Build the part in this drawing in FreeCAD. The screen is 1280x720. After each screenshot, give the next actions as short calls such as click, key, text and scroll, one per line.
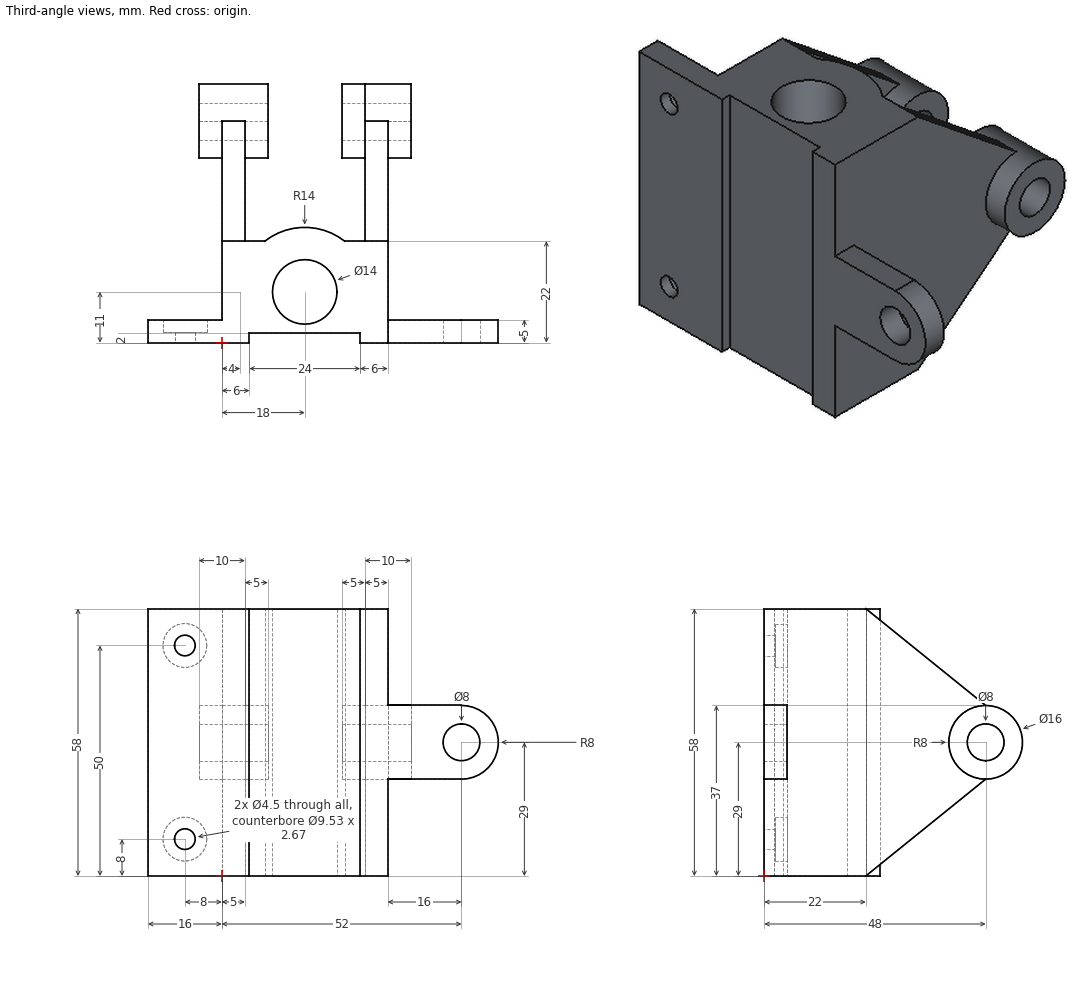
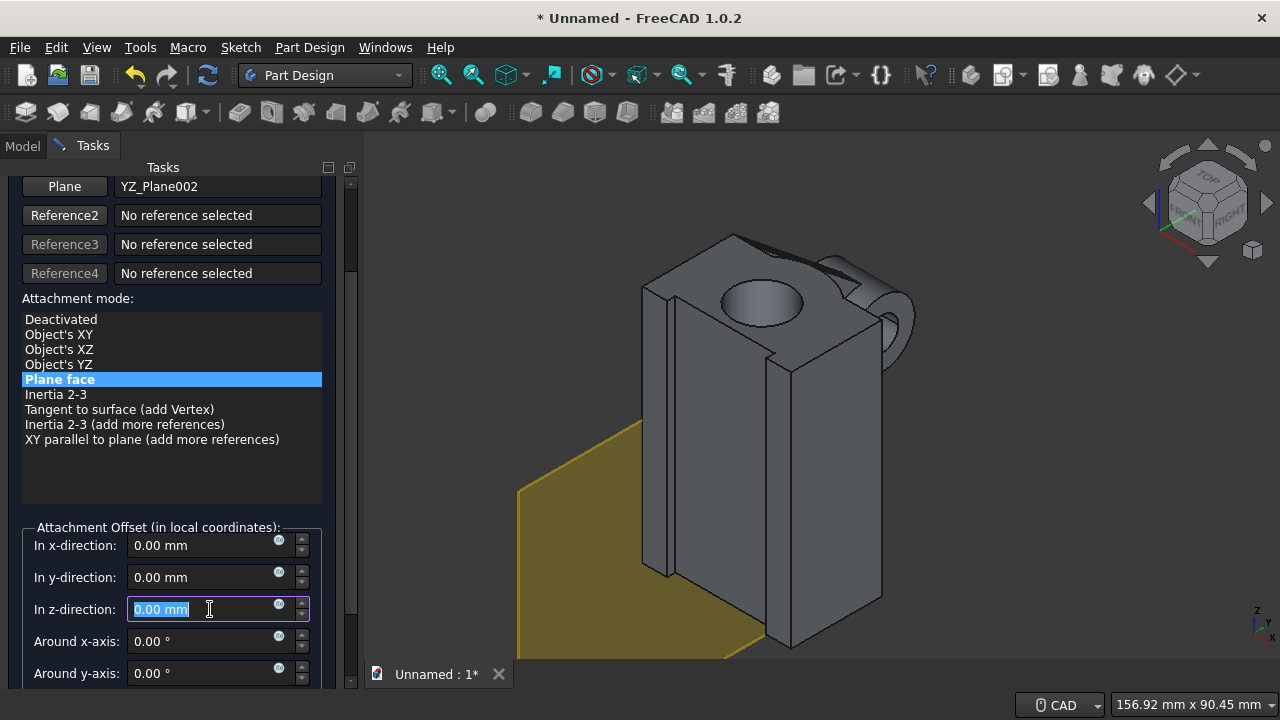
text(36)
key(Tab)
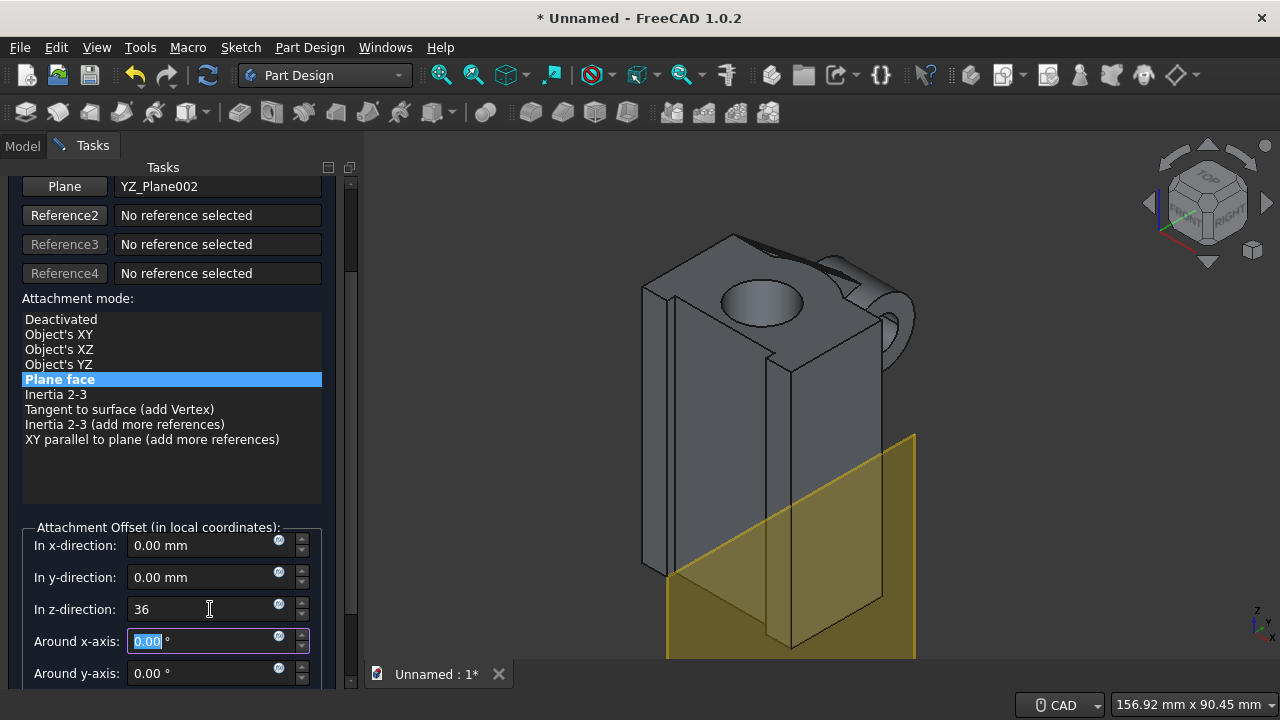
scroll(351, 432, up, 3)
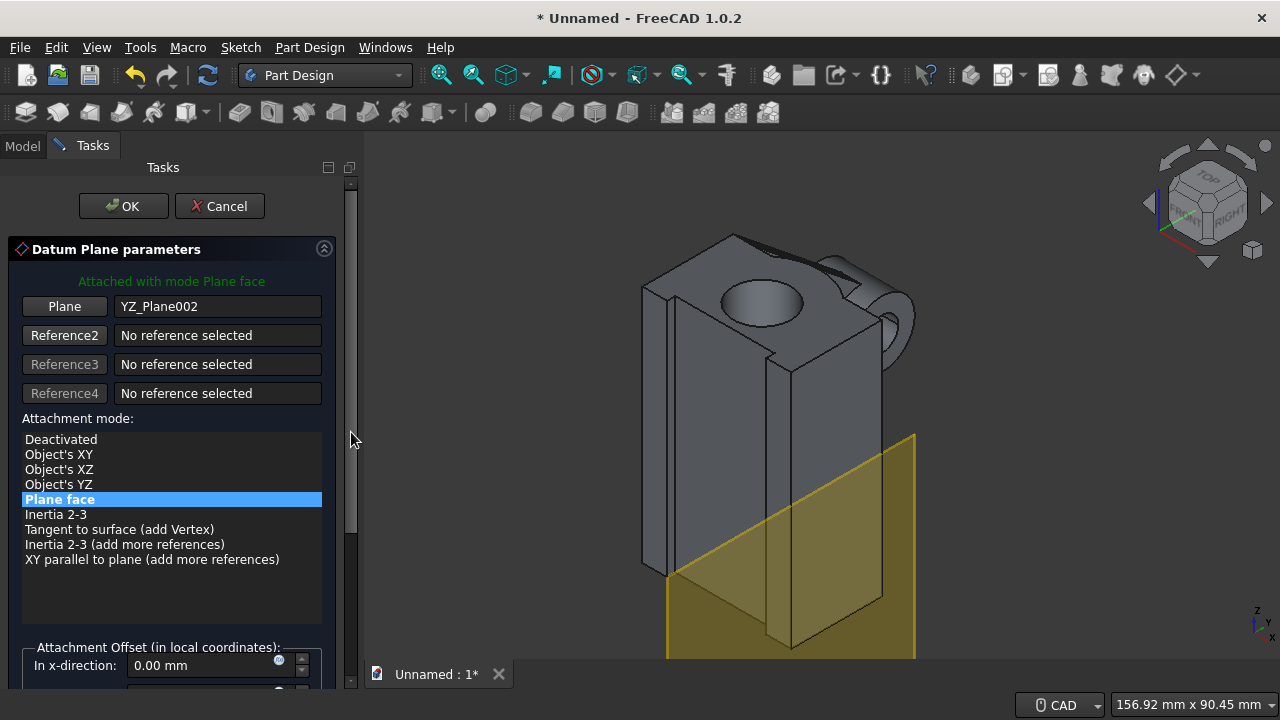
click(124, 206)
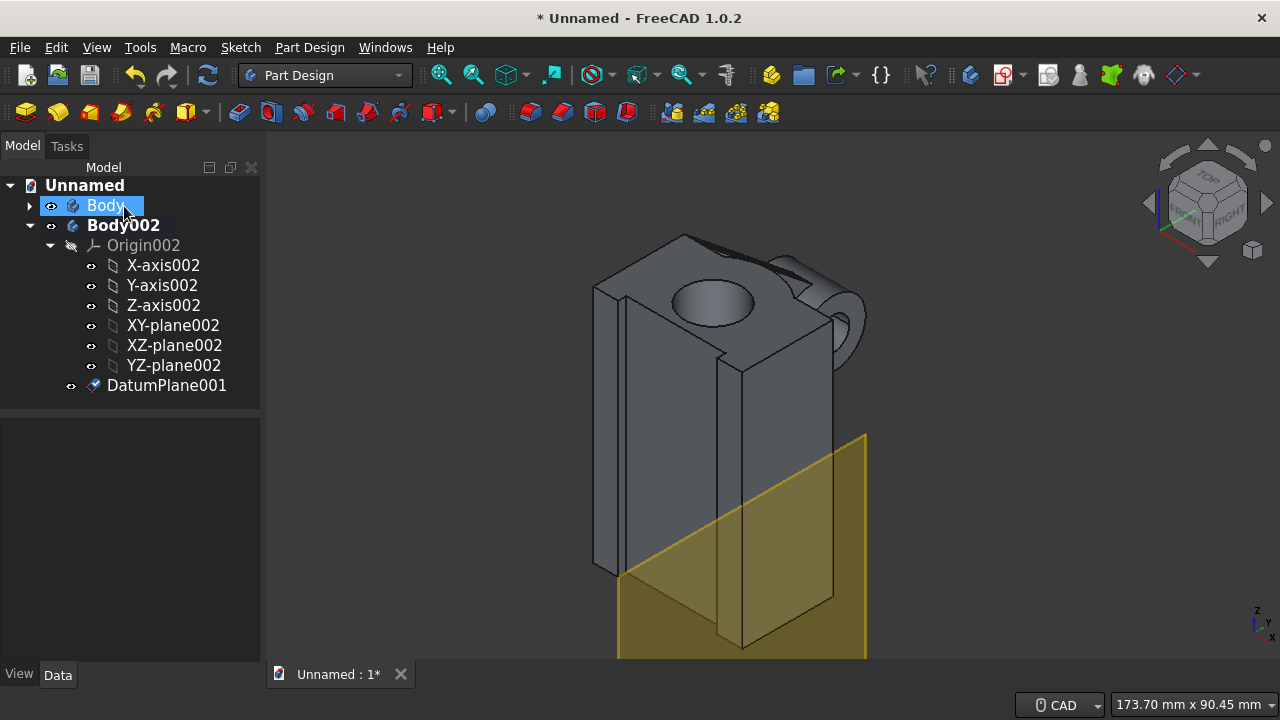
click(116, 386)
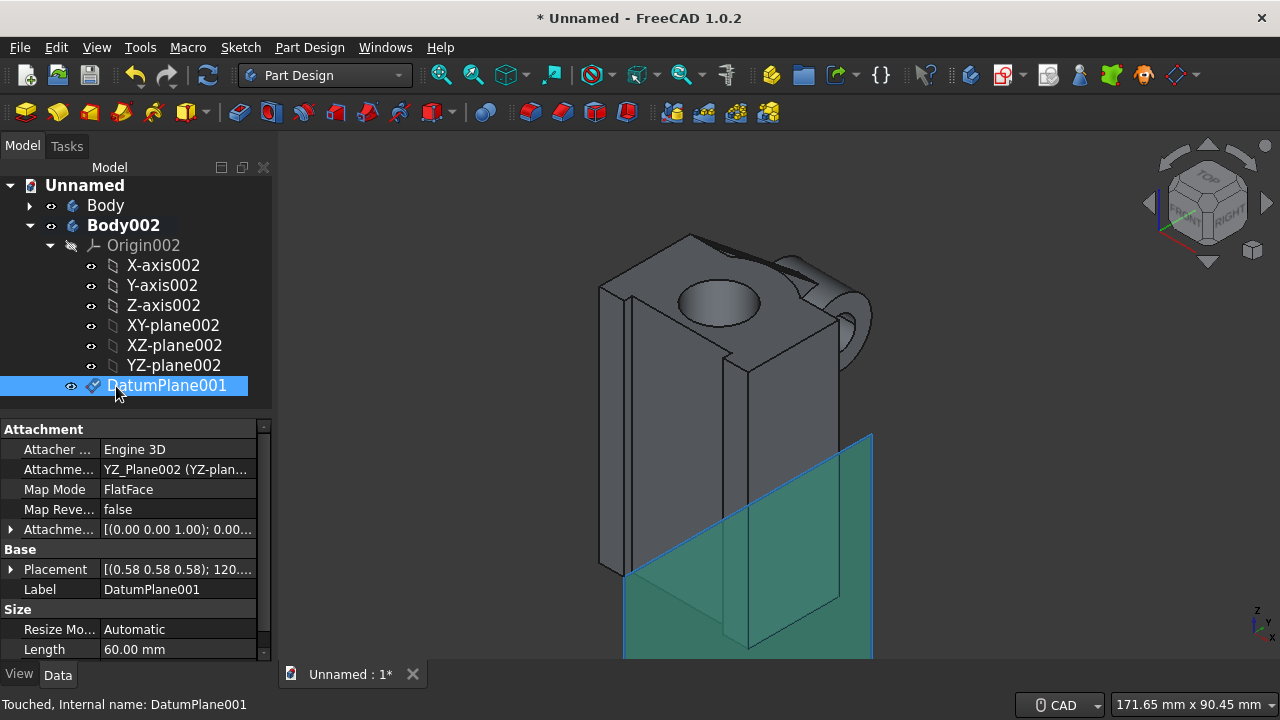
click(1004, 76)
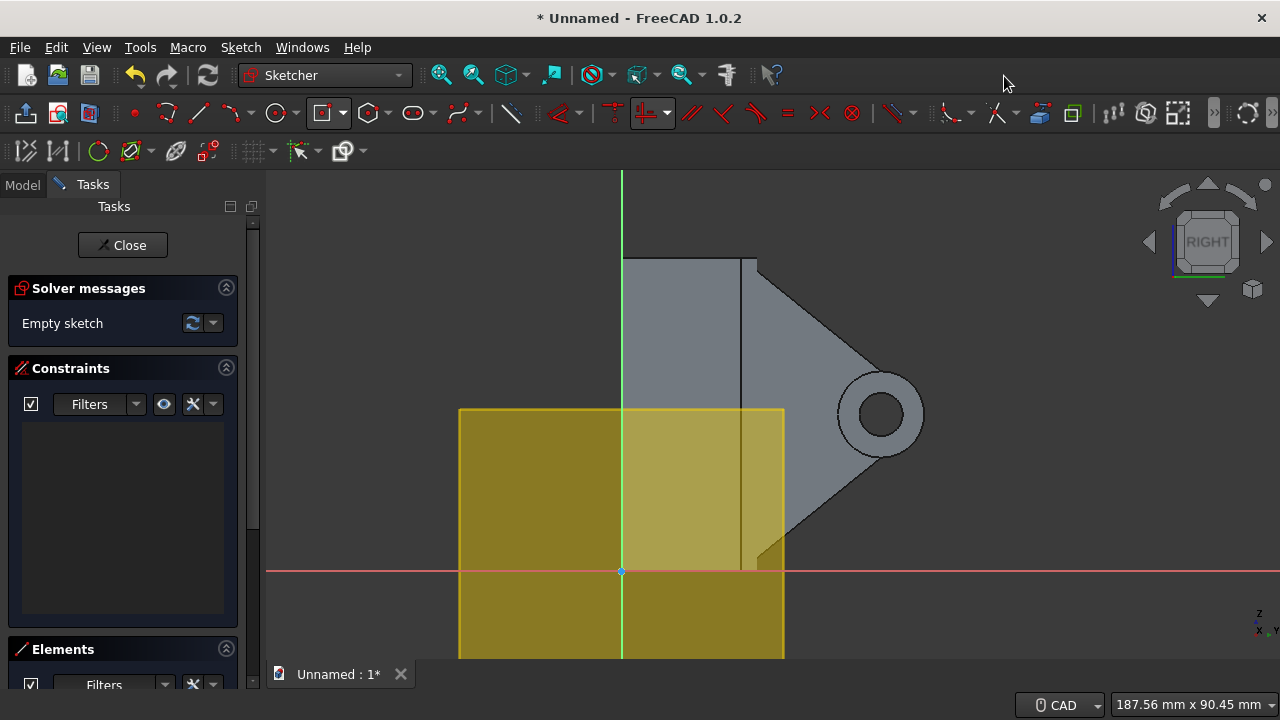
scroll(957, 415, up, 6)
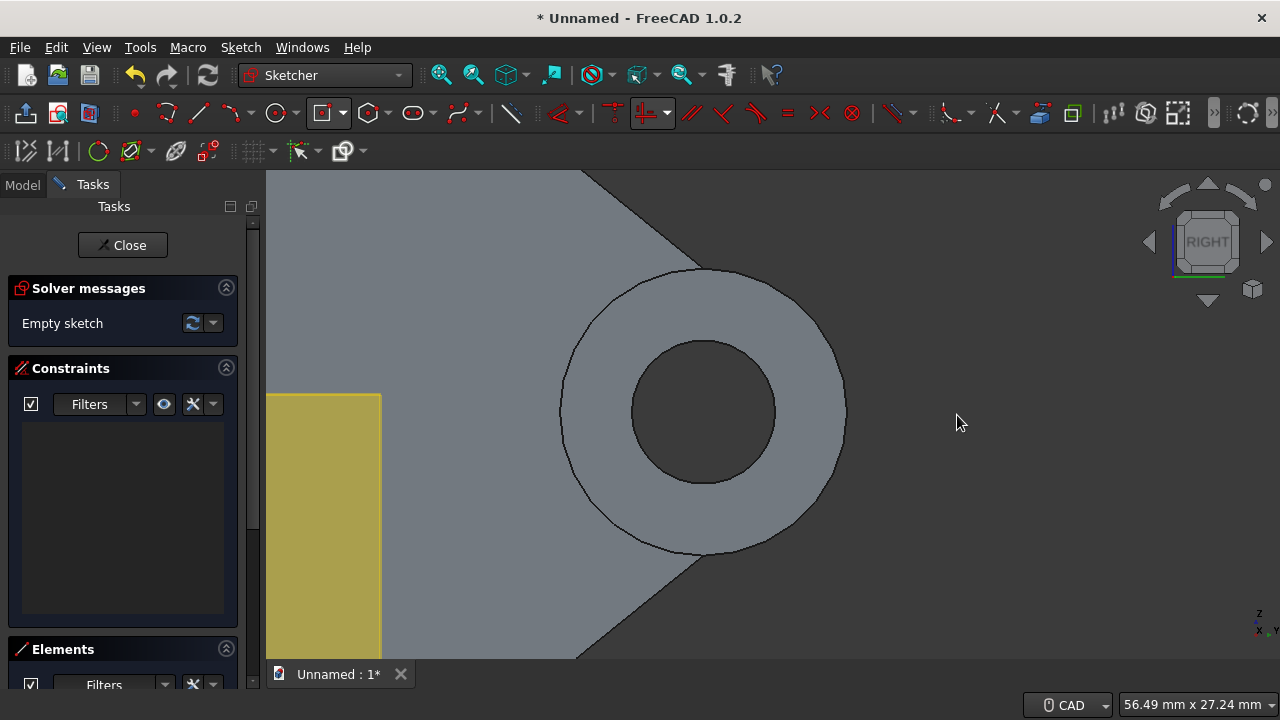
key(g)
key(c)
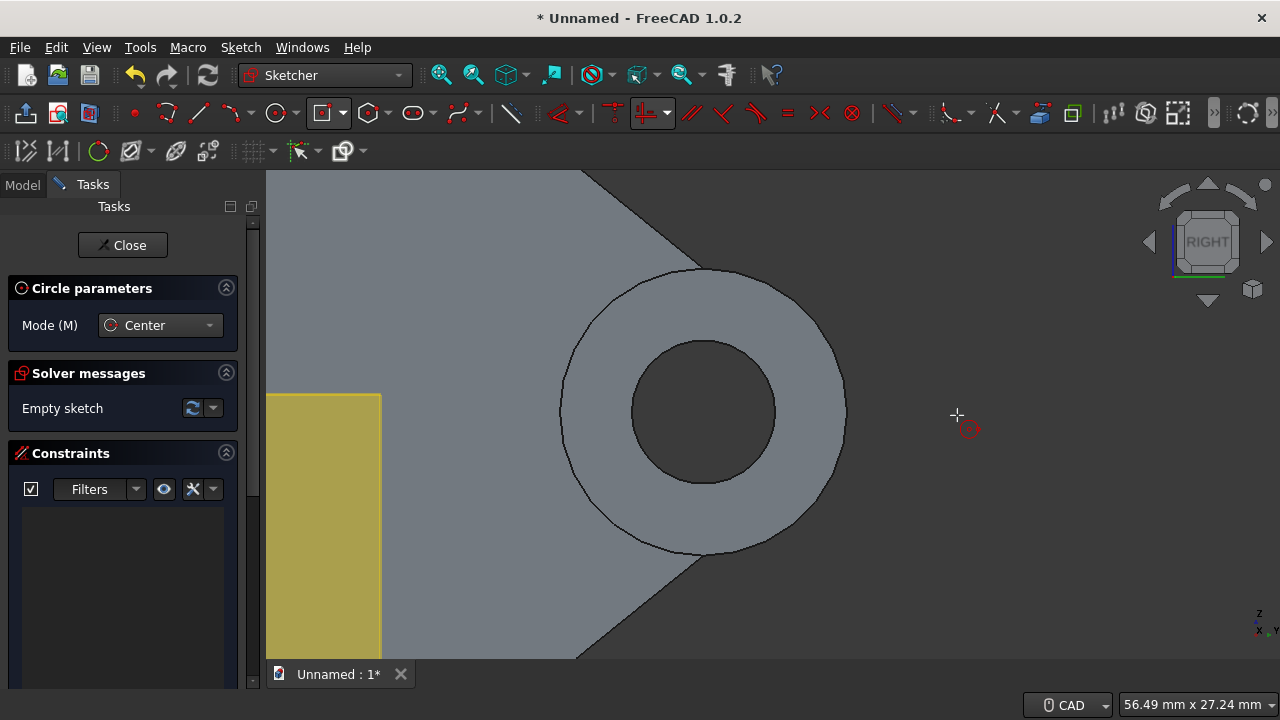
click(704, 412)
move(805, 311)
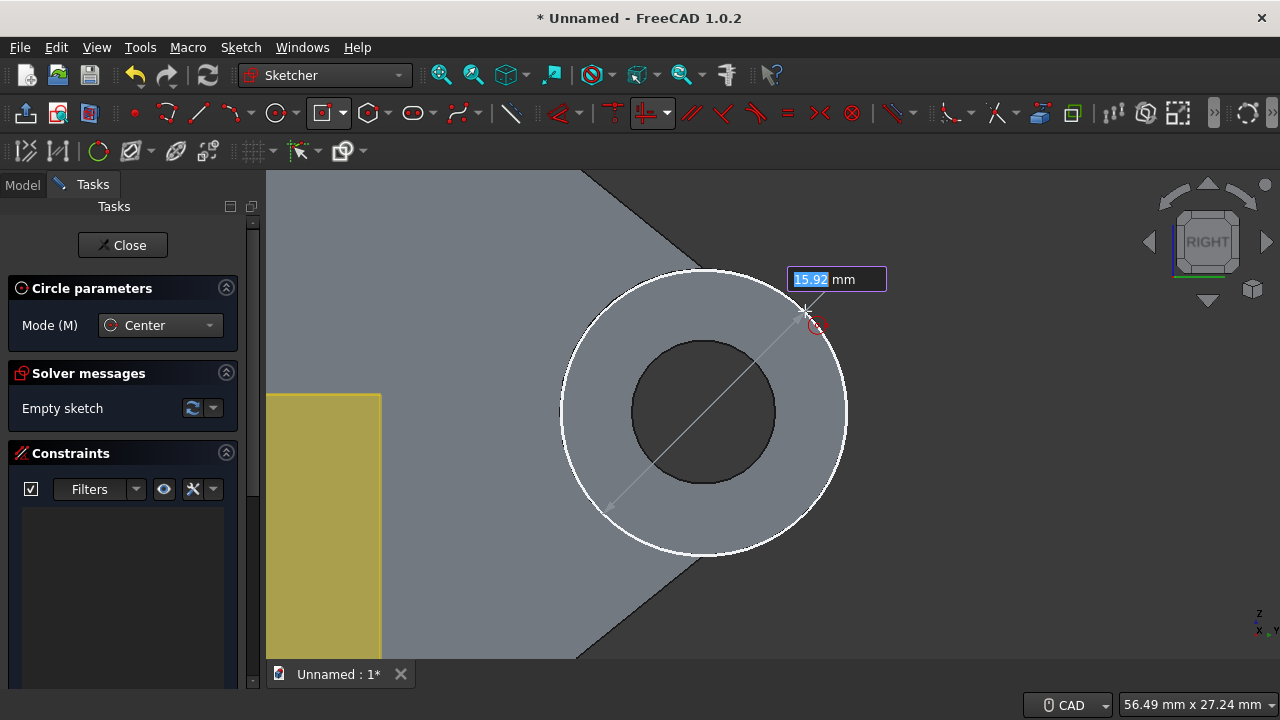
text(16)
key(Return)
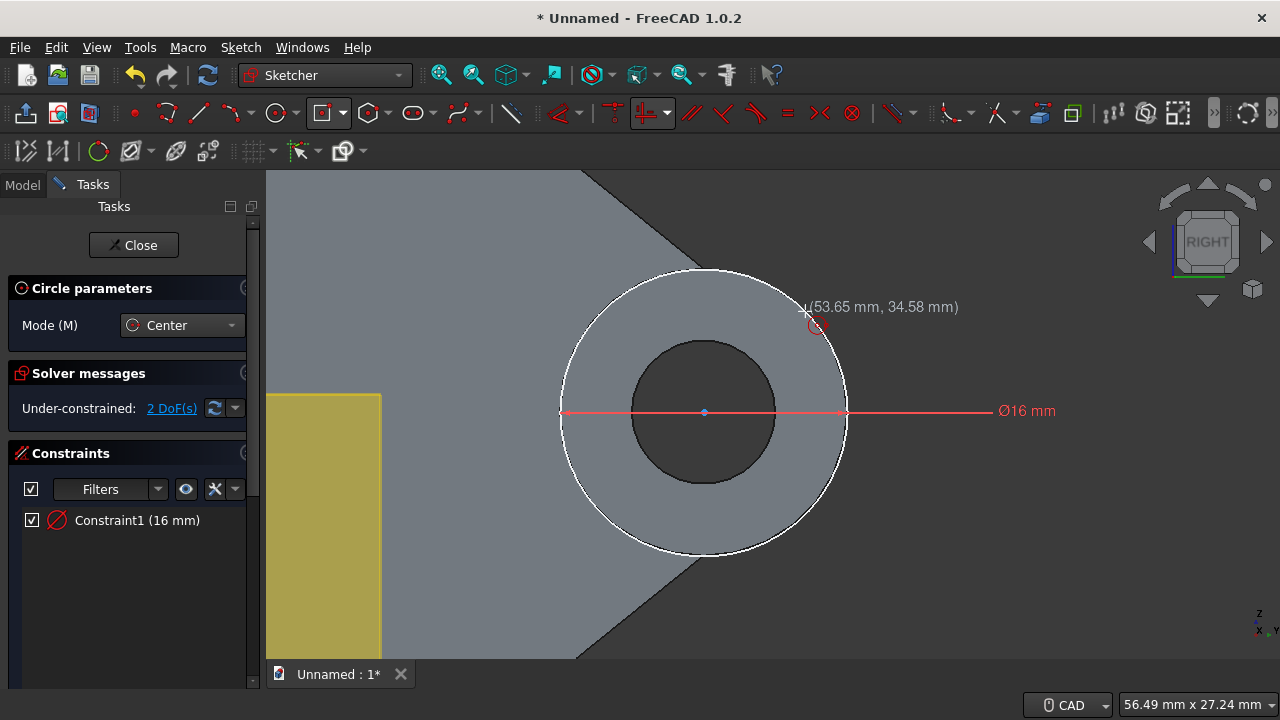
click(704, 413)
move(754, 361)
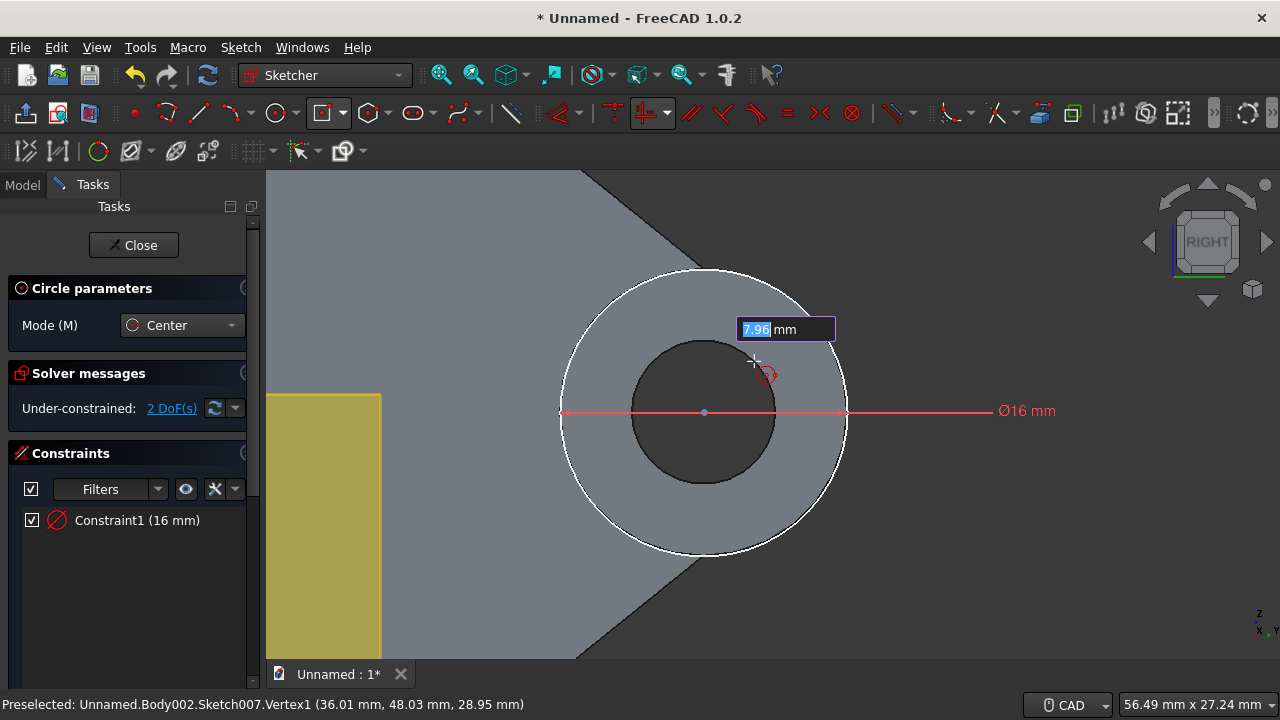
text(8)
key(Return)
key(Escape)